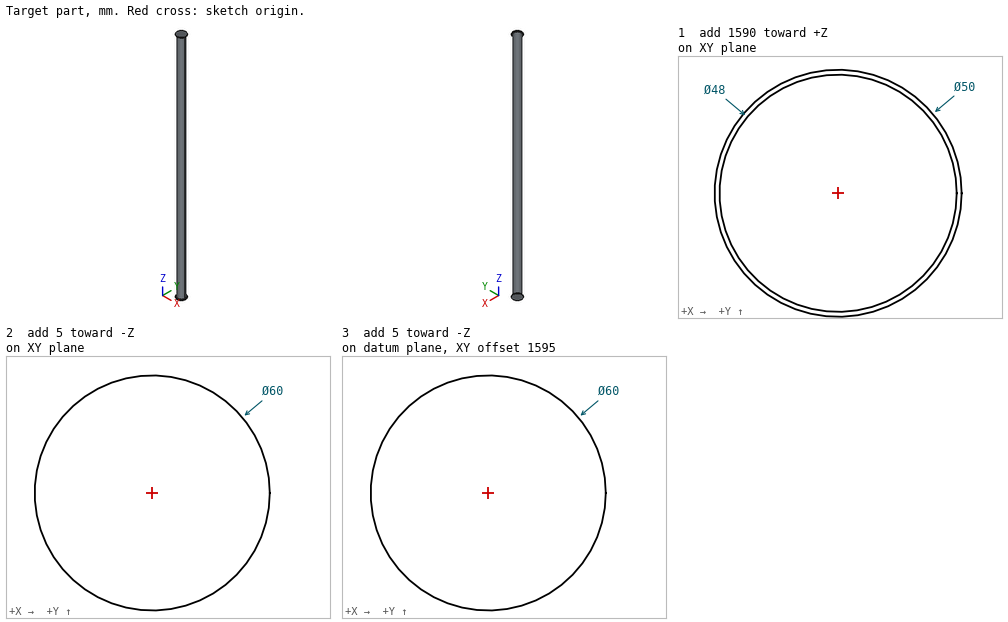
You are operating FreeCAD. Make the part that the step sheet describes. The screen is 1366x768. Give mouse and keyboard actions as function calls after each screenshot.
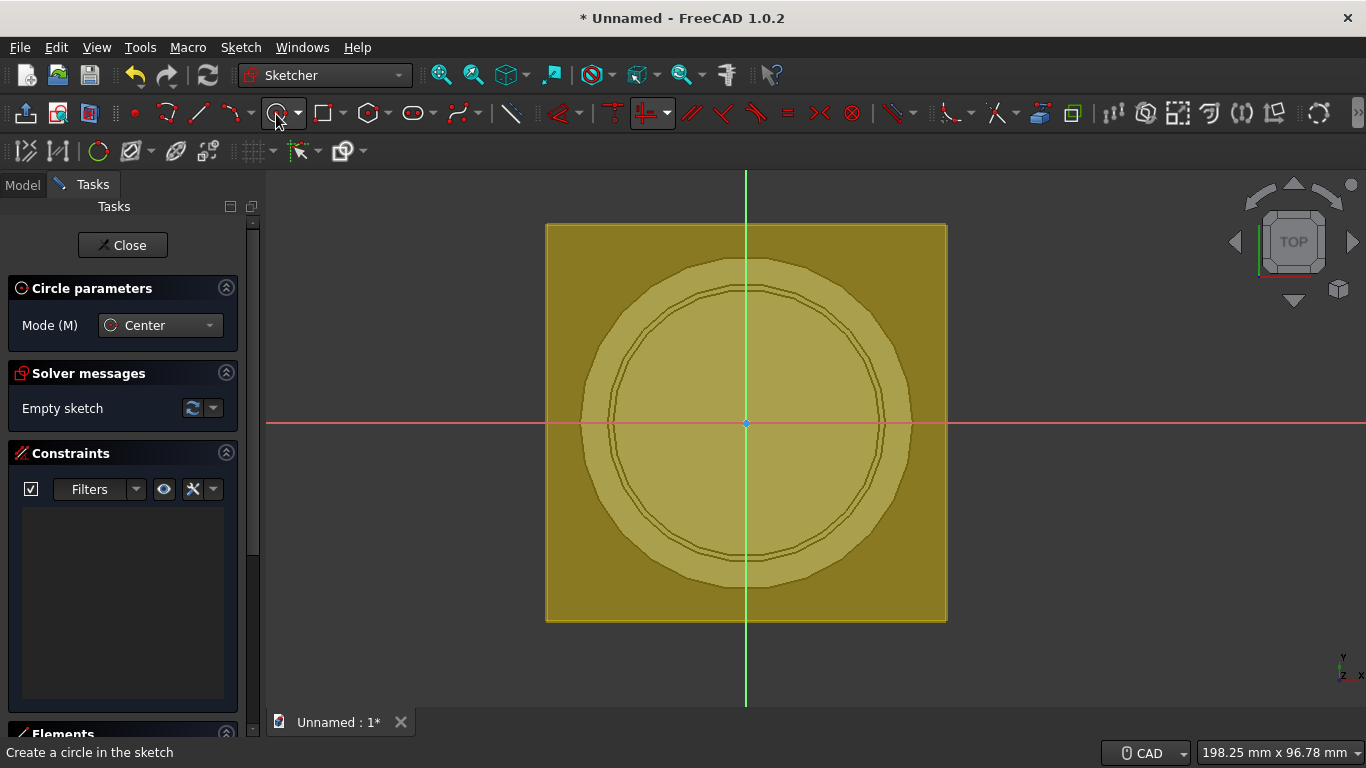
click(746, 423)
move(864, 305)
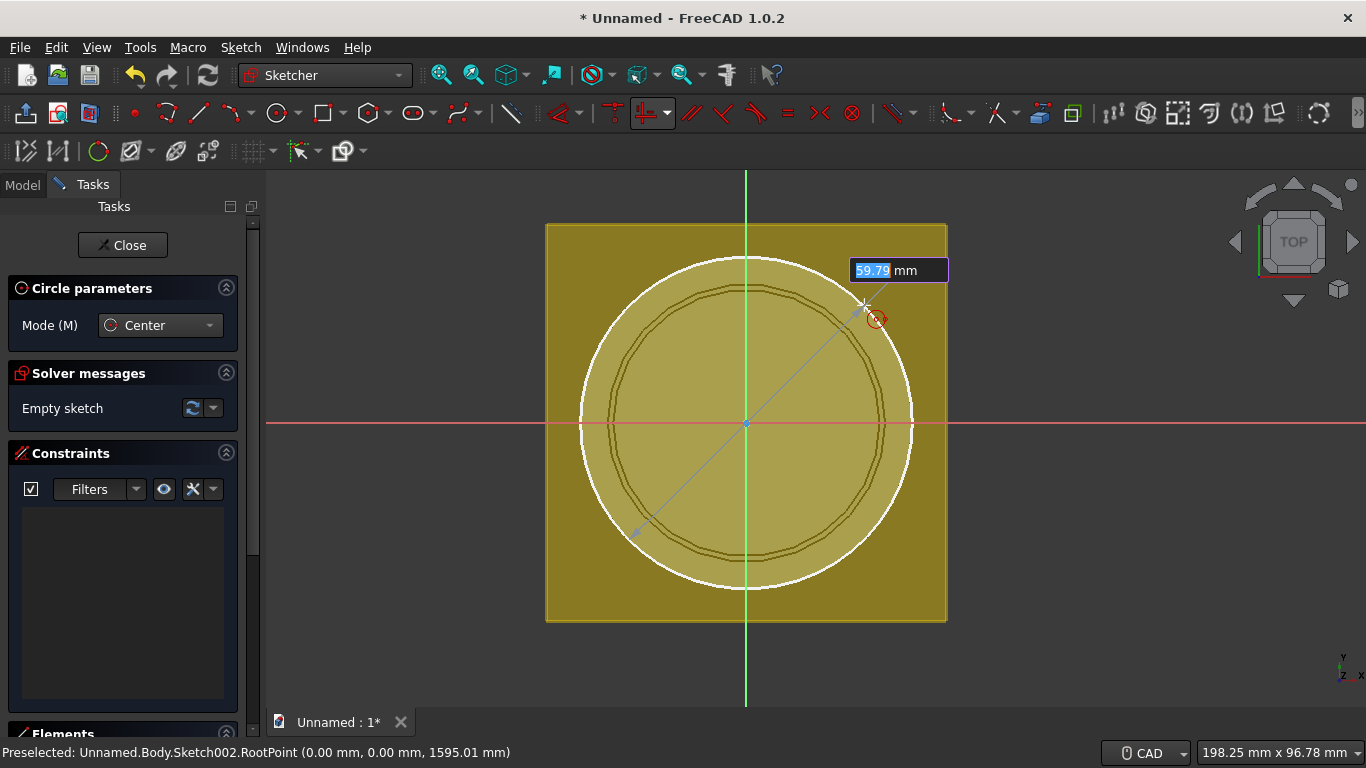
text(60)
key(Return)
key(Escape)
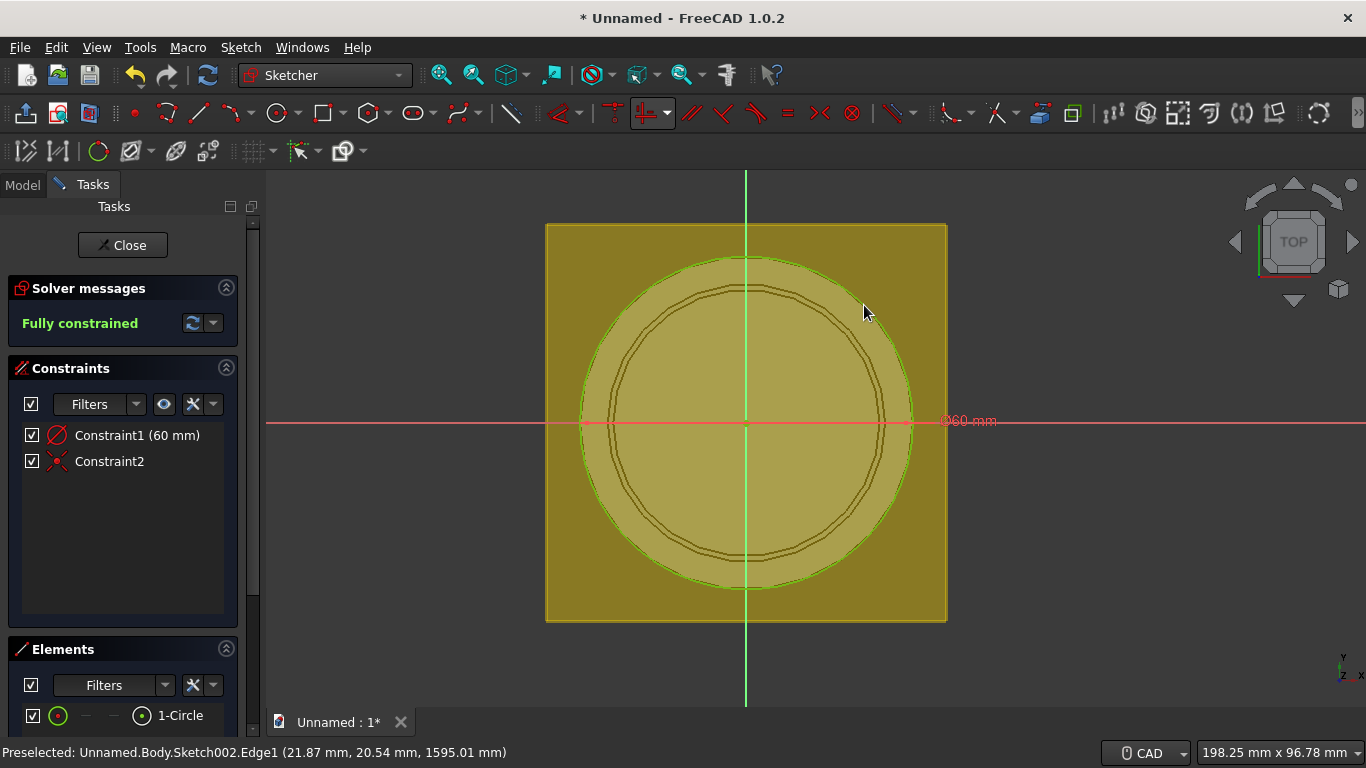
click(123, 245)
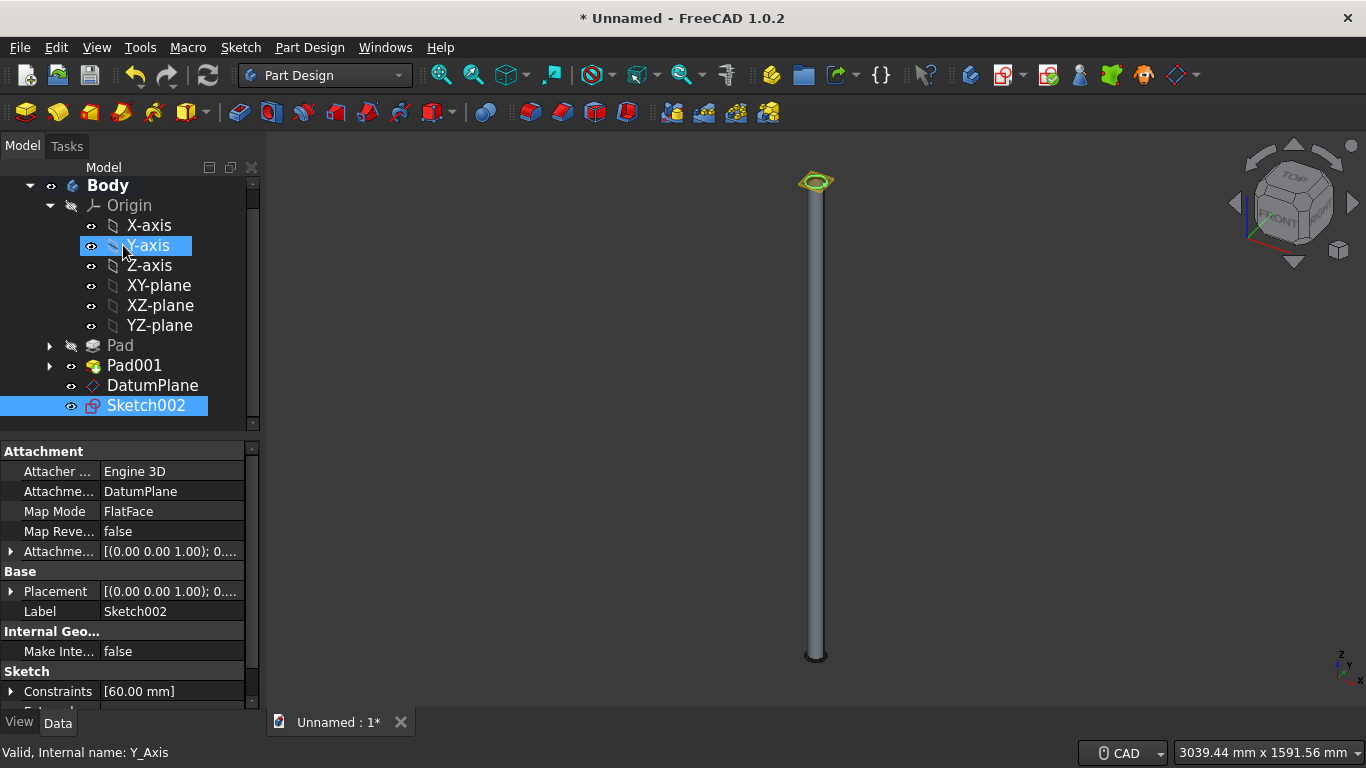
click(26, 112)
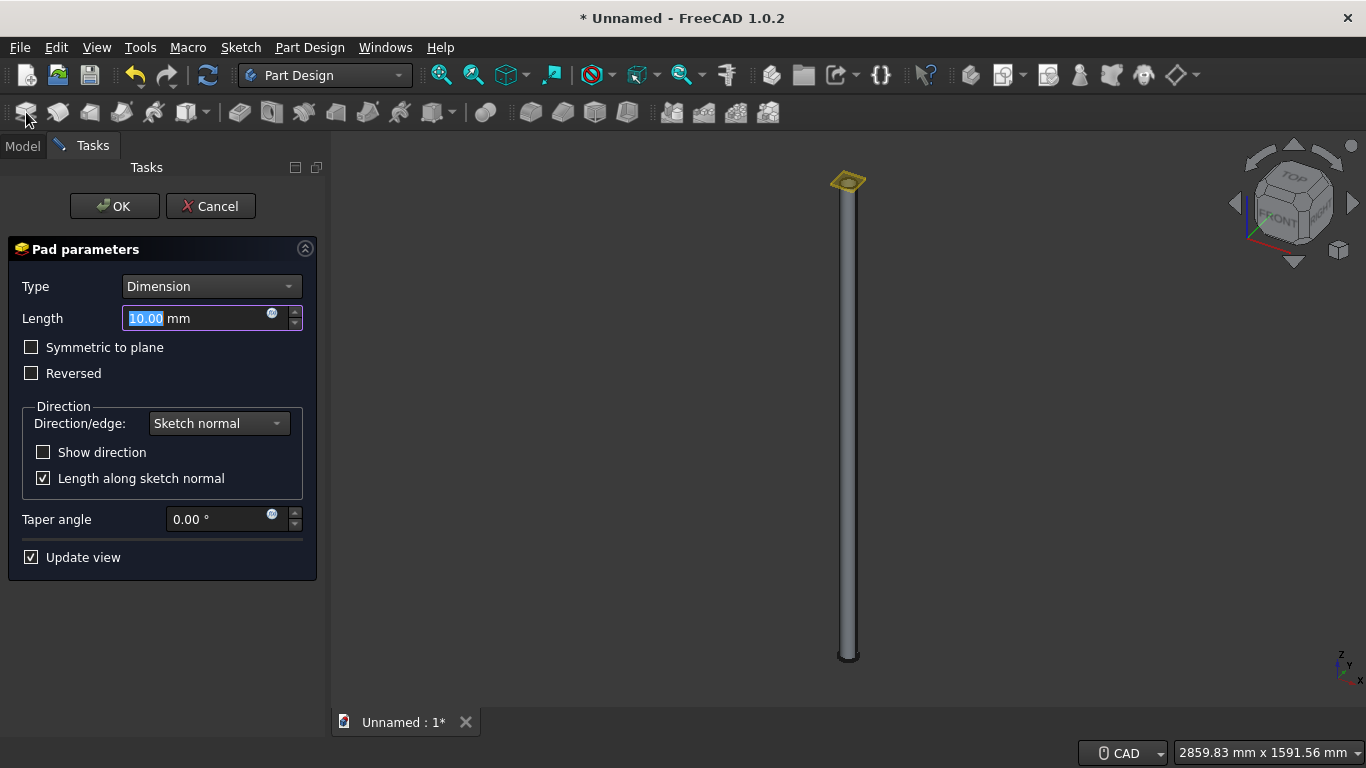
text(5)
key(Tab)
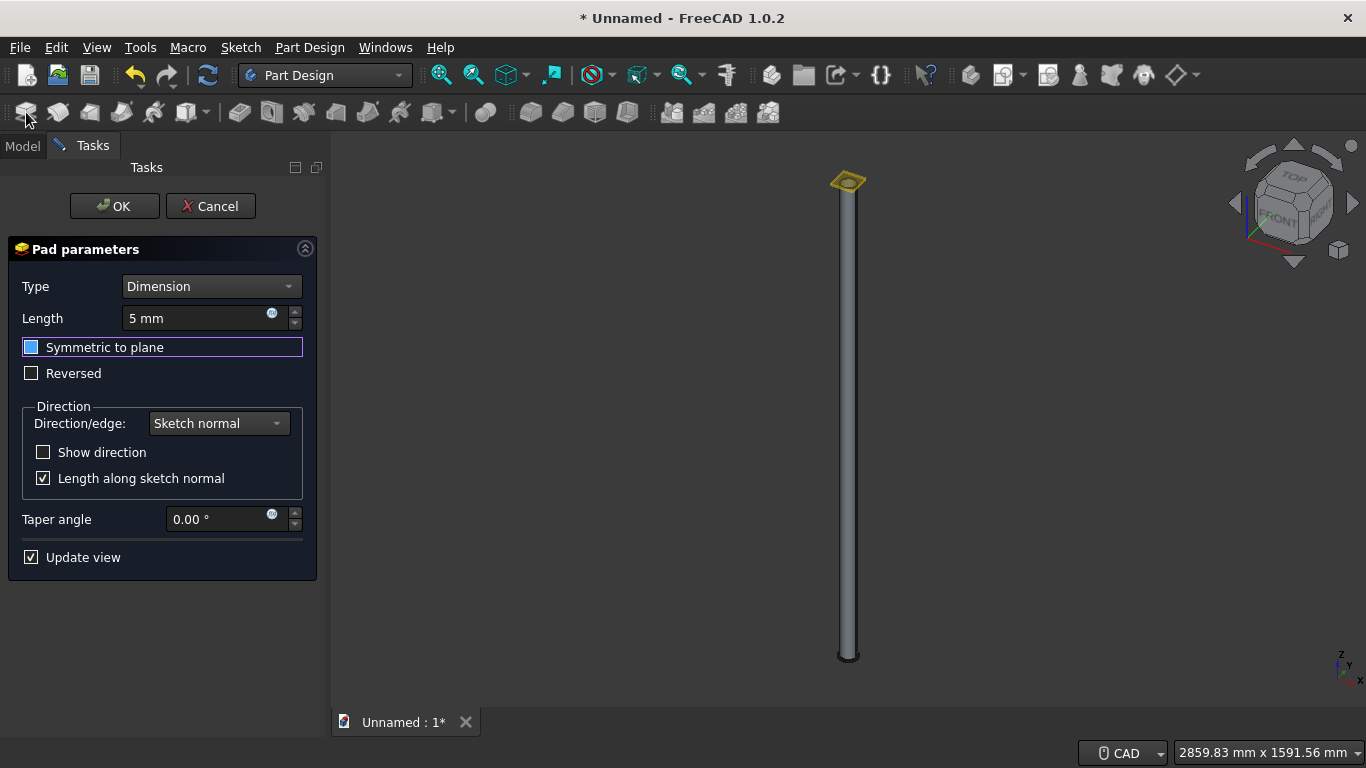
click(30, 373)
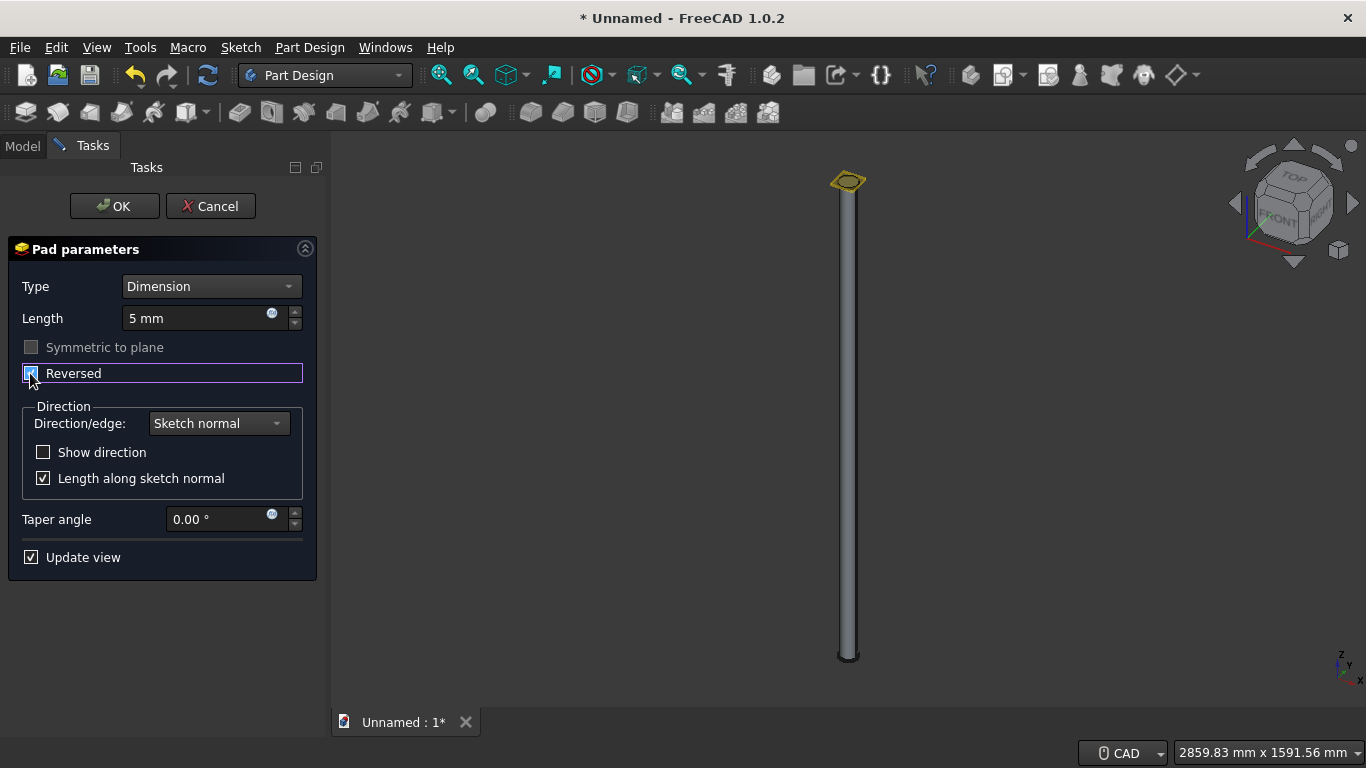
click(115, 206)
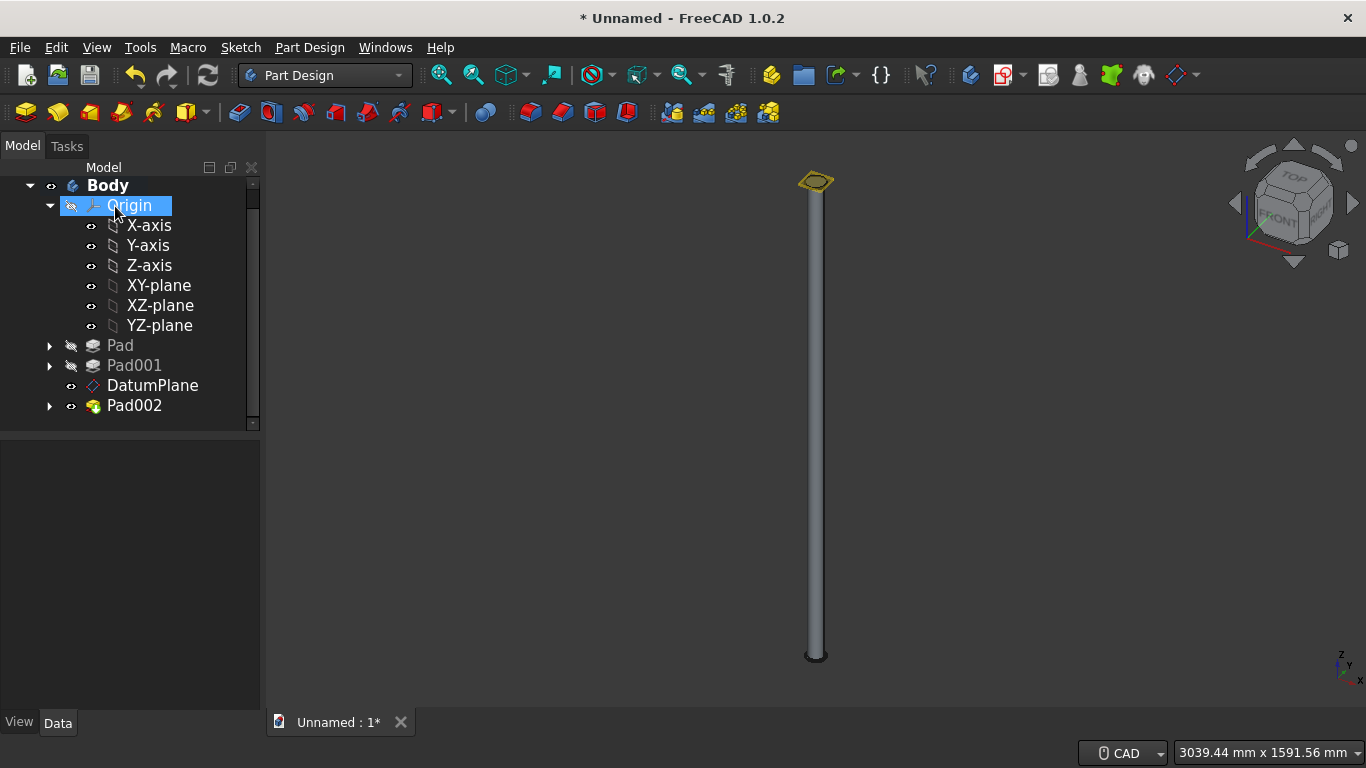
click(116, 386)
key(space)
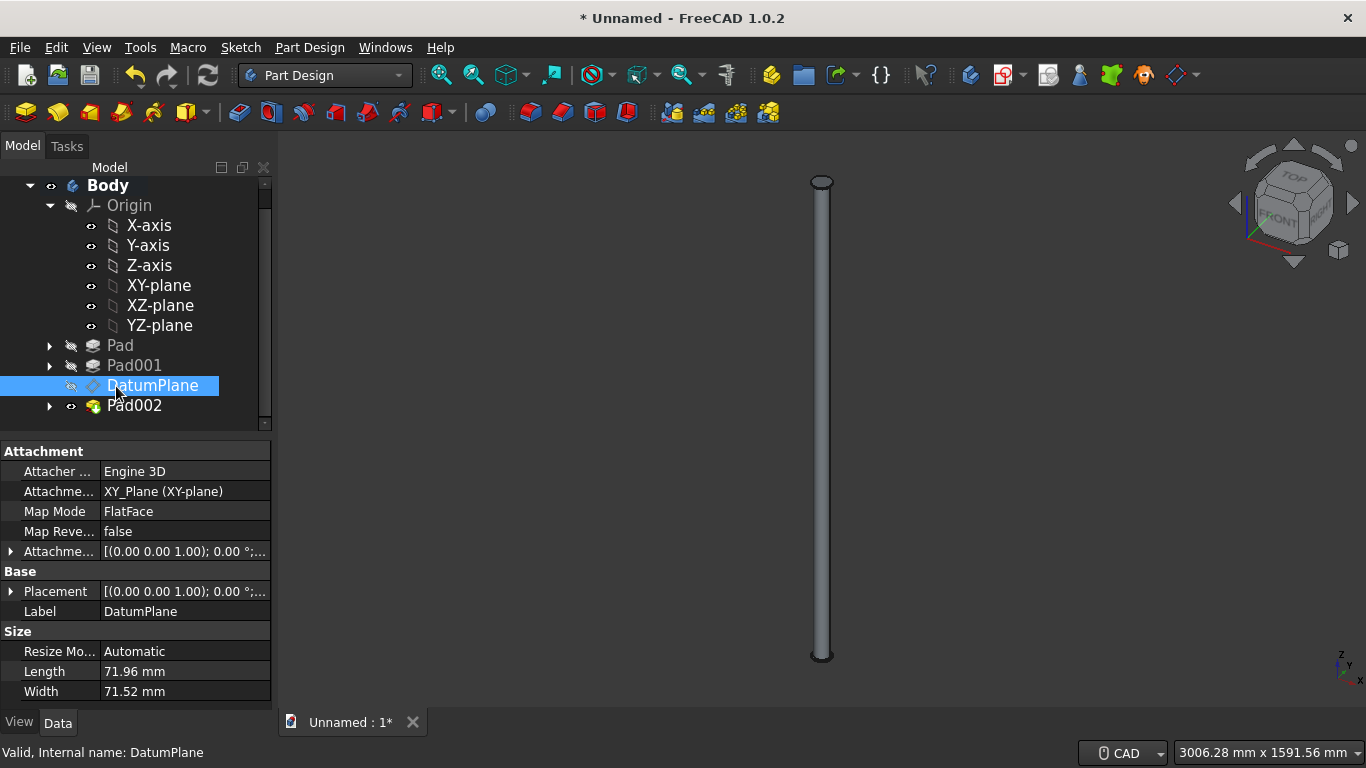
key(0)